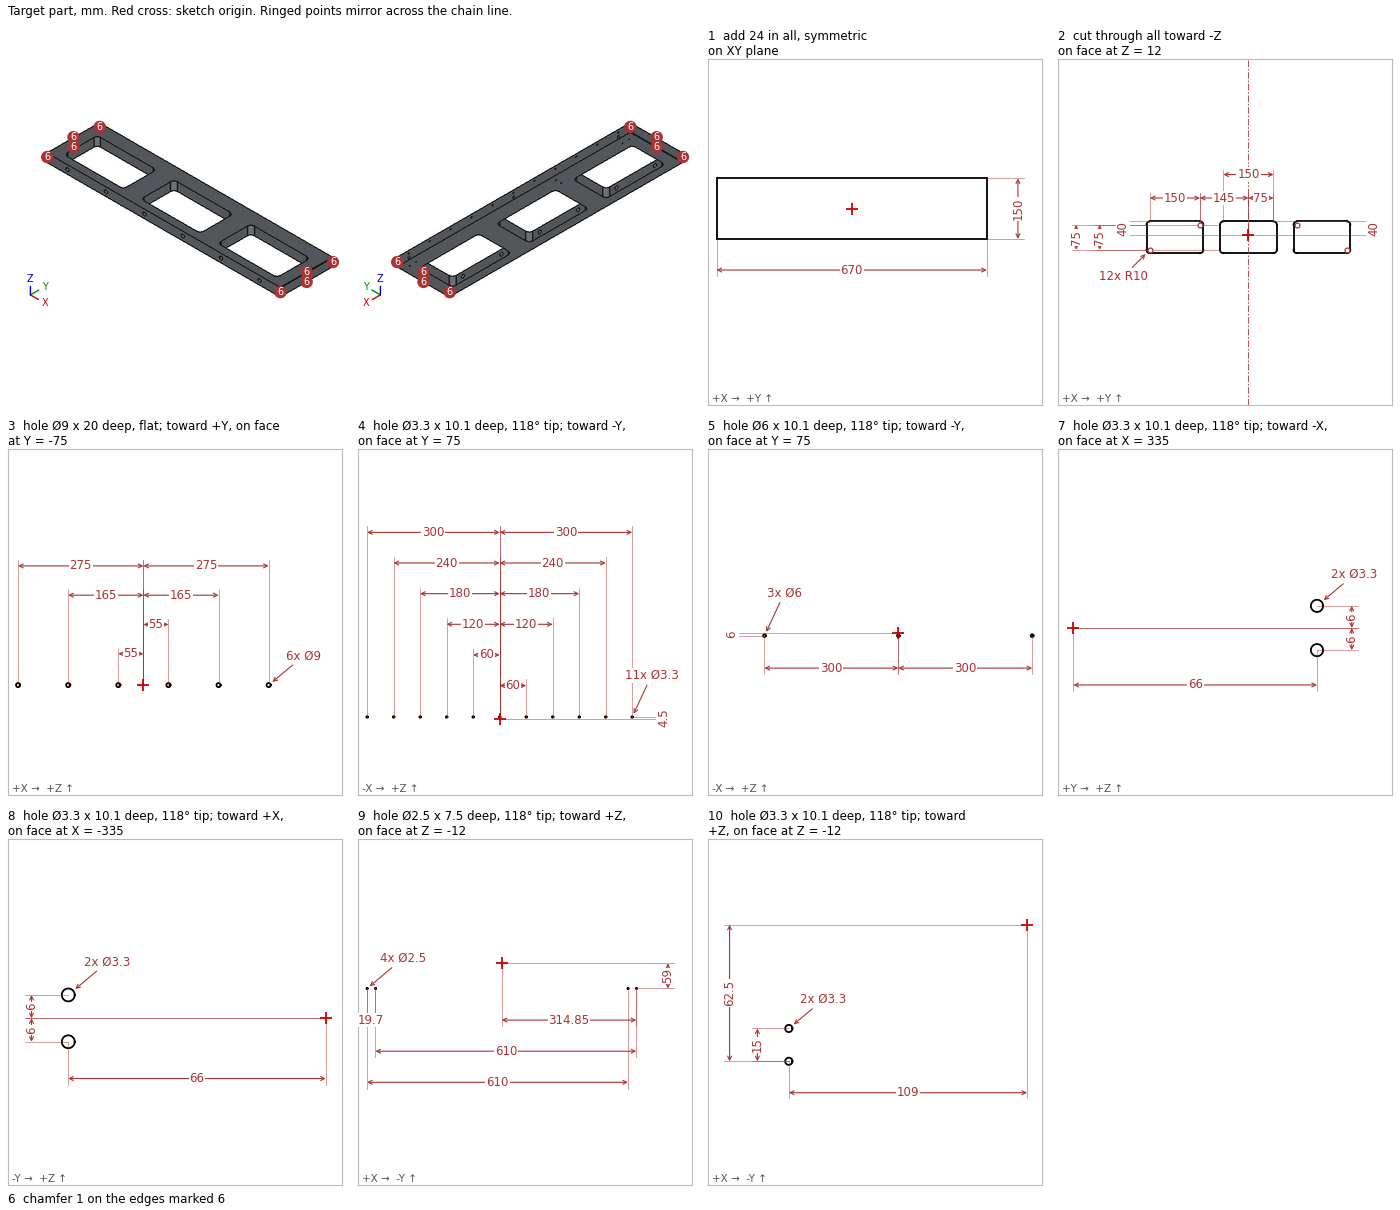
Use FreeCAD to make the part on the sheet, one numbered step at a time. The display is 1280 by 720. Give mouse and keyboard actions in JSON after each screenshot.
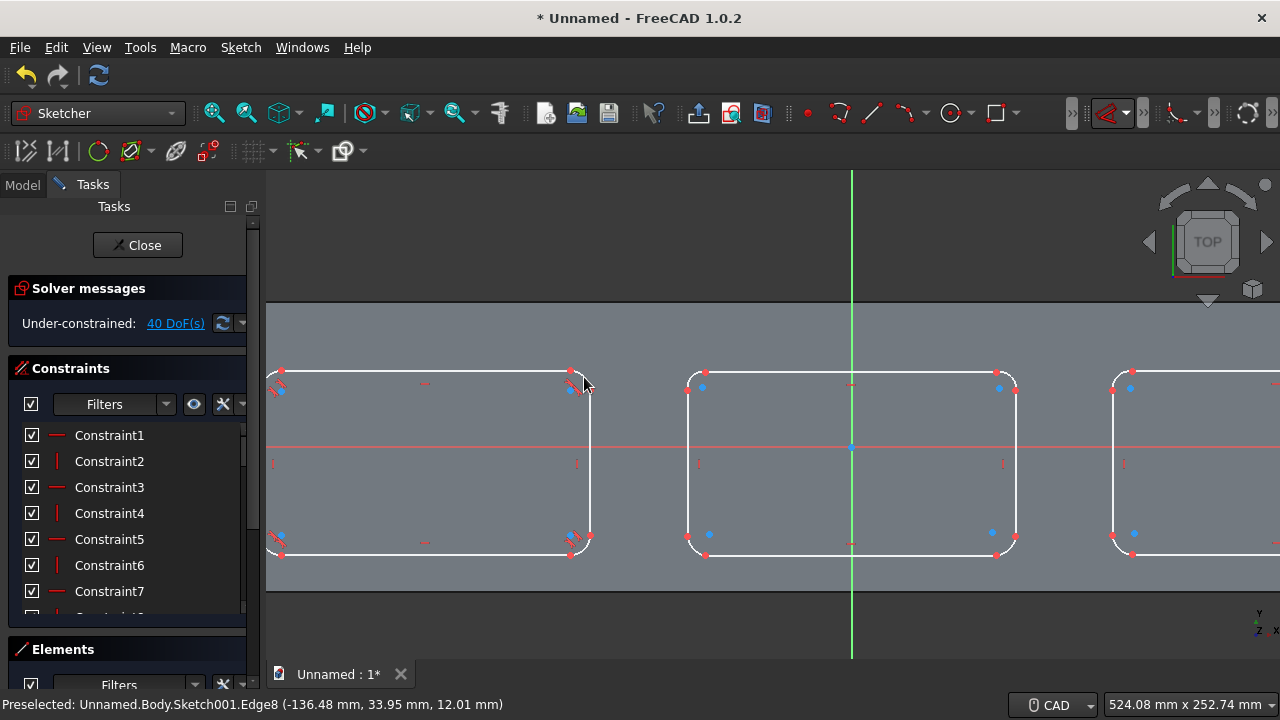
{"action": "left_click", "coordinate": [909, 372]}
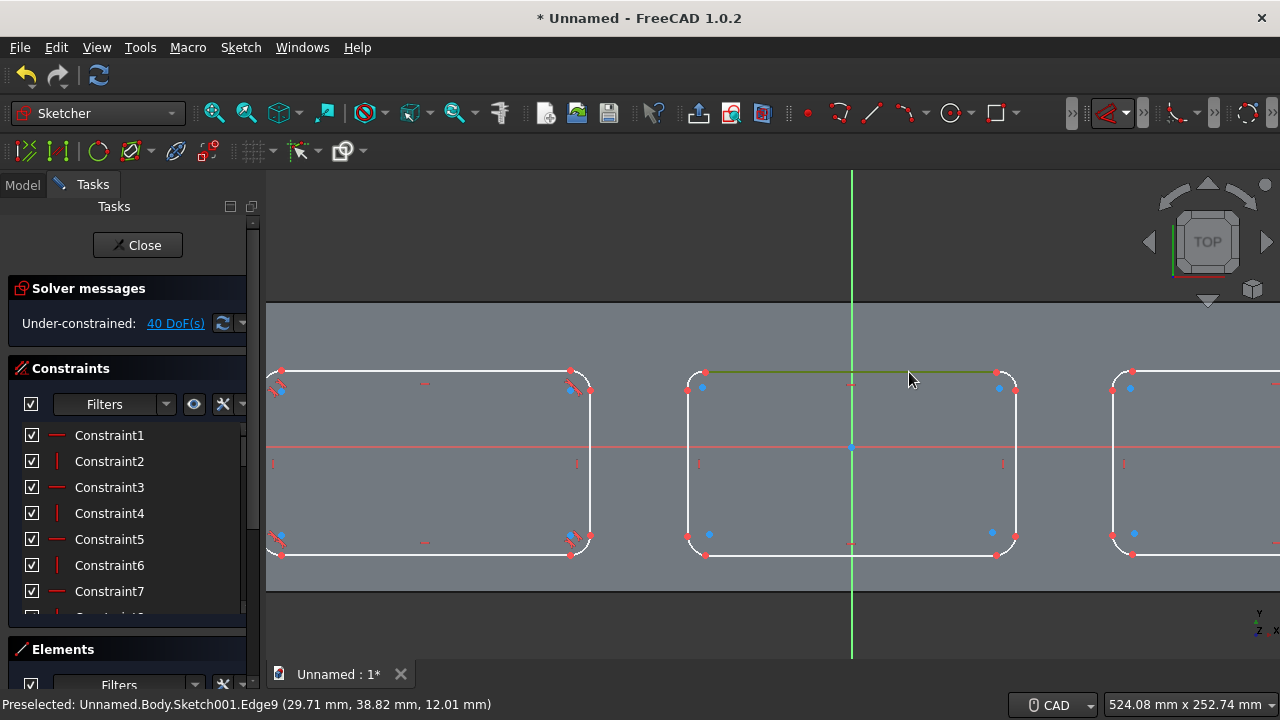
{"action": "left_click", "coordinate": [692, 377]}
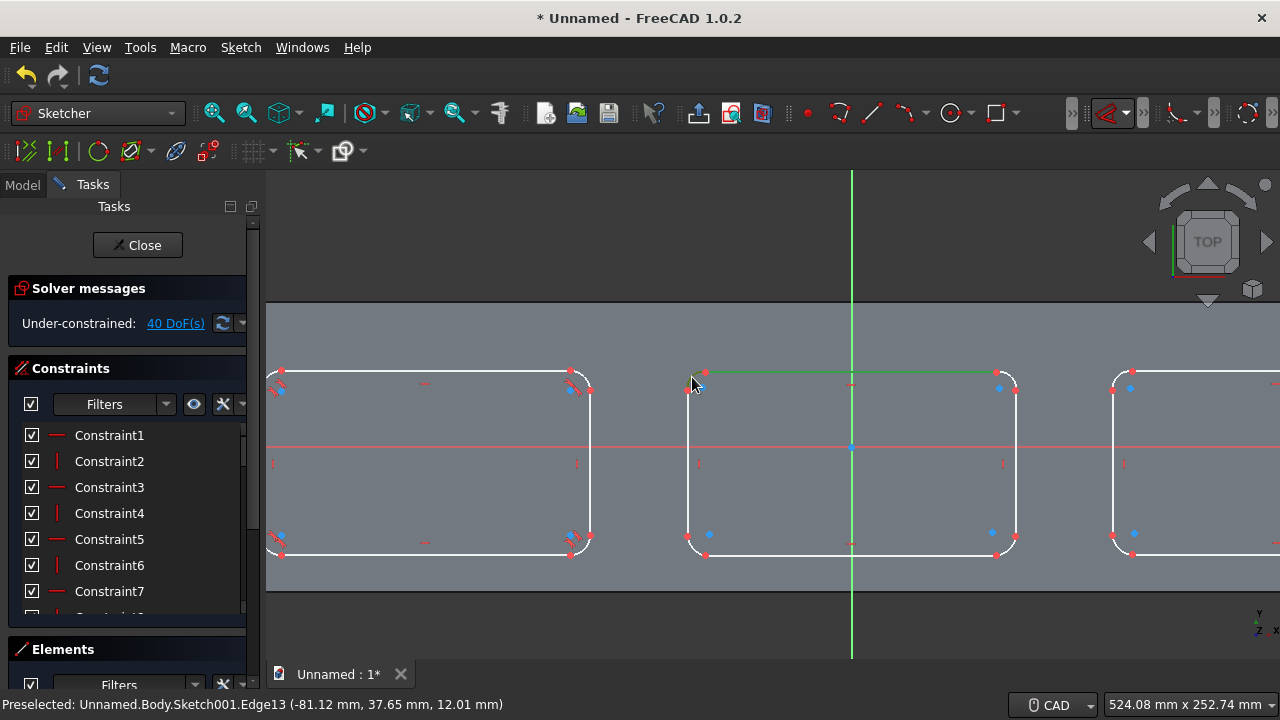
{"action": "key", "text": "t"}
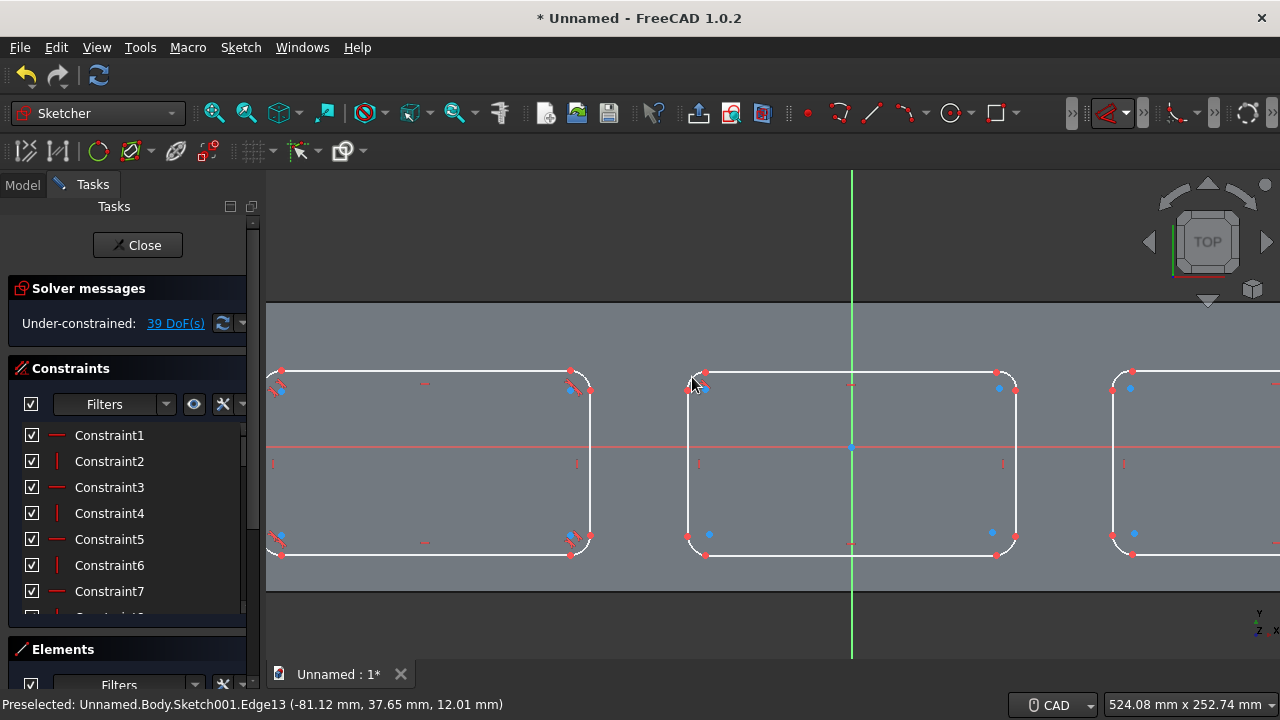
{"action": "left_click", "coordinate": [909, 372]}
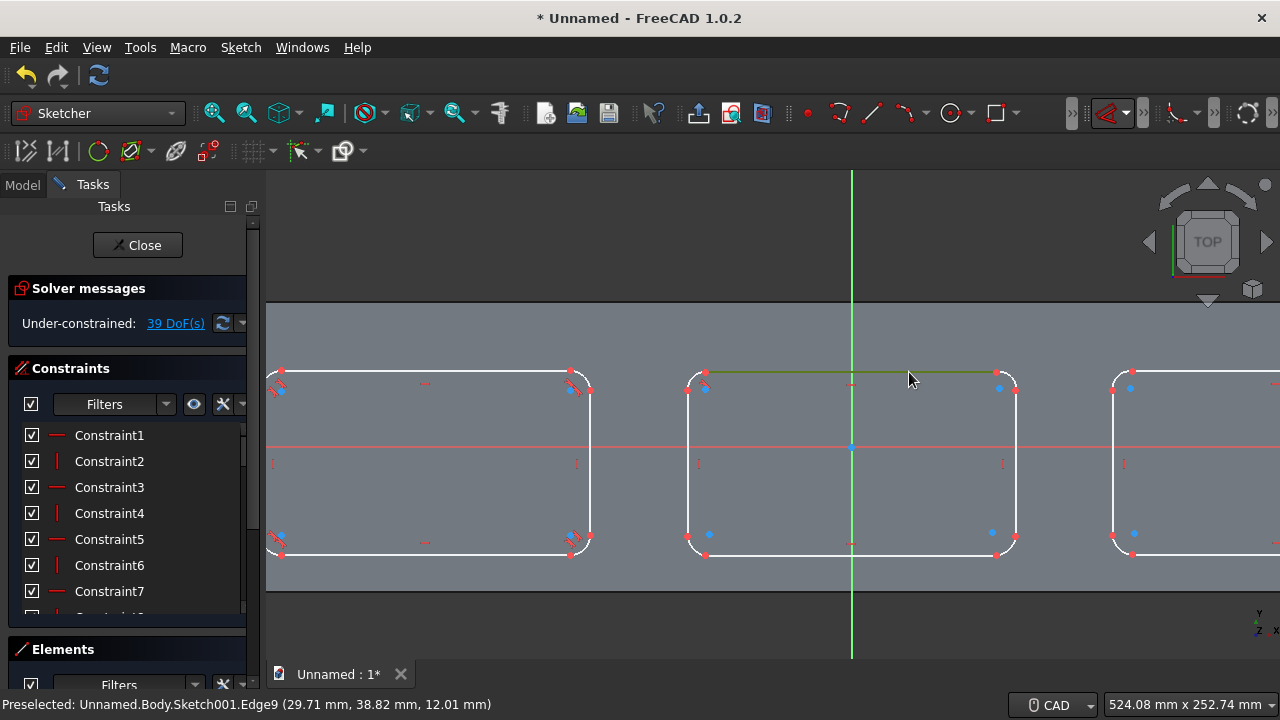
{"action": "left_click", "coordinate": [1011, 376]}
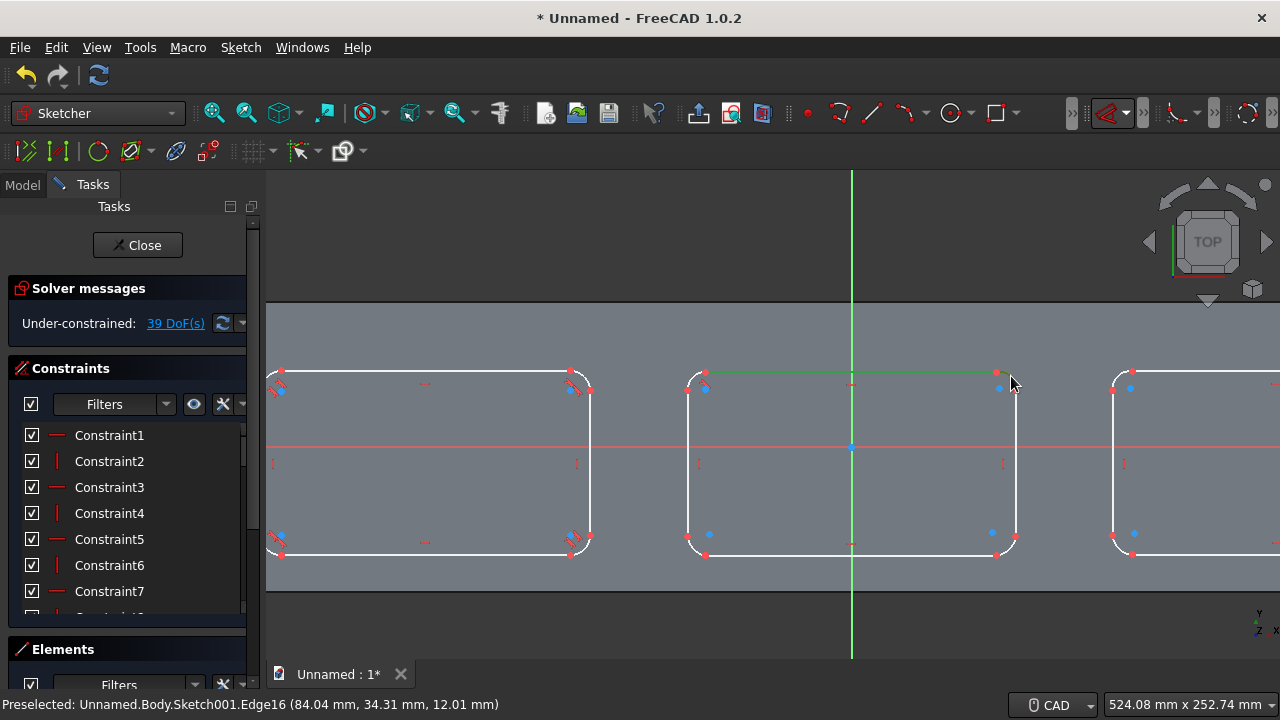
{"action": "key", "text": "t"}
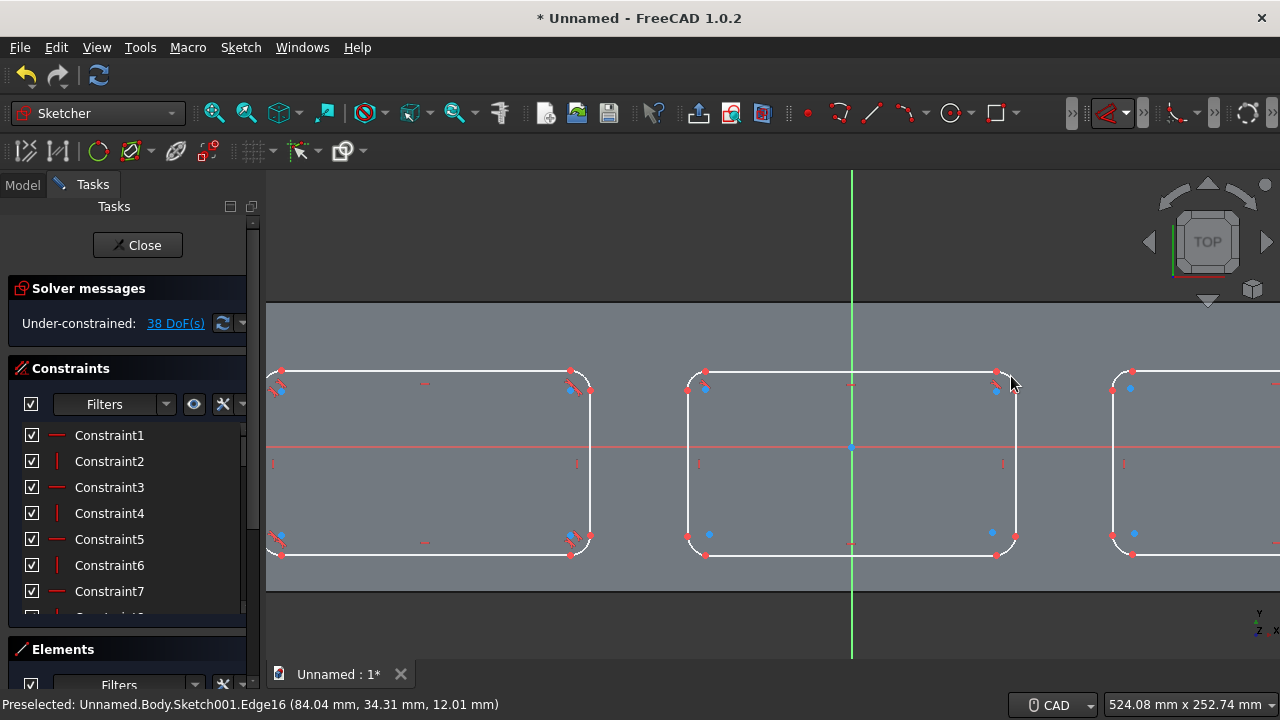
{"action": "left_click", "coordinate": [688, 434]}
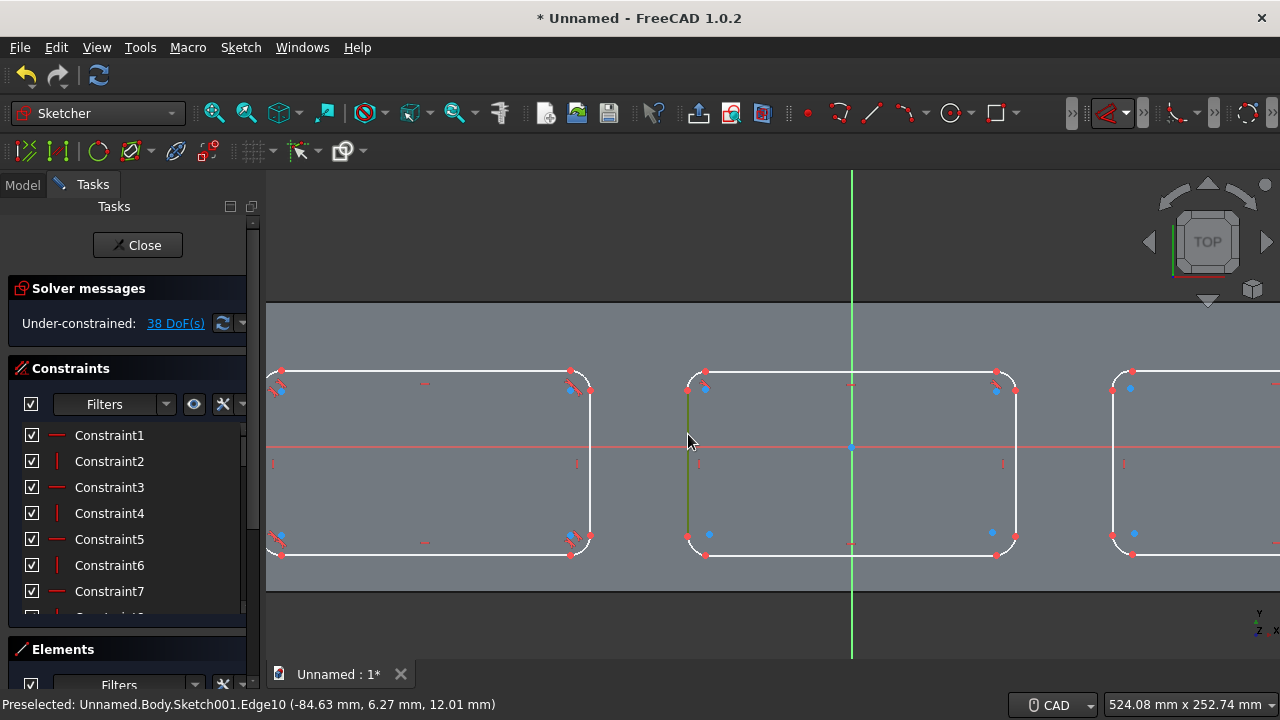
{"action": "left_click", "coordinate": [693, 377]}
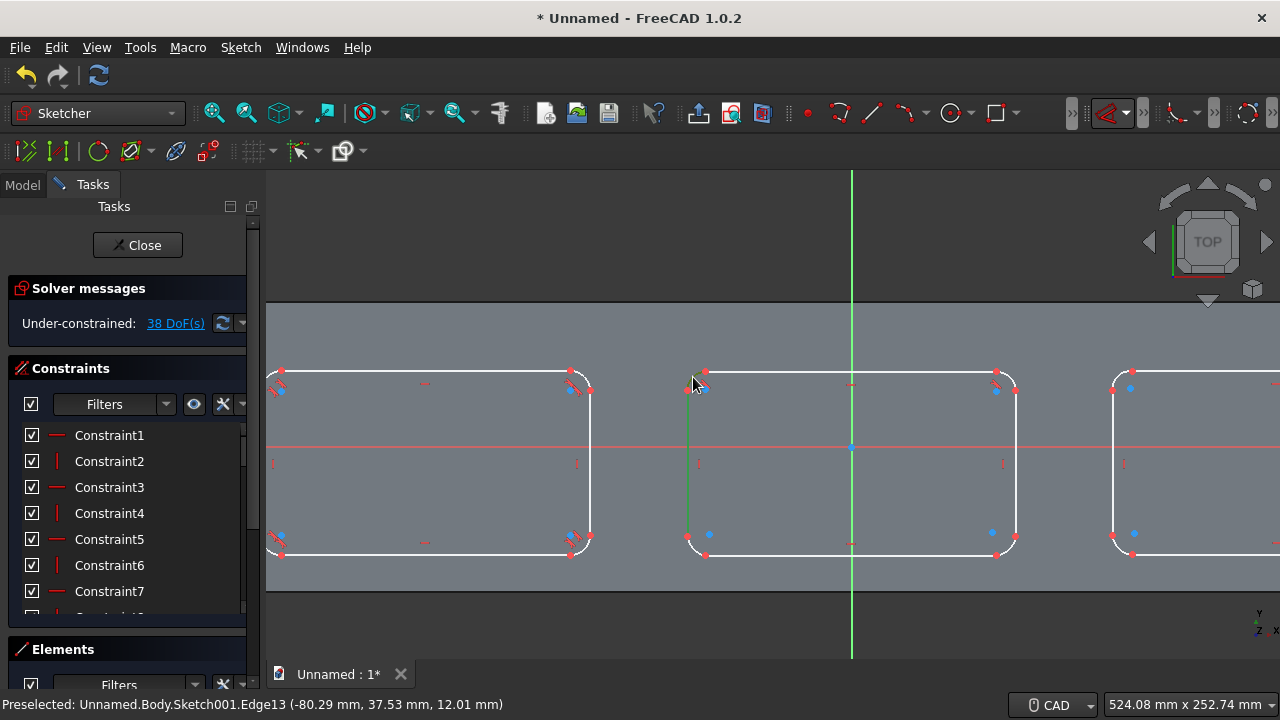
{"action": "key", "text": "t"}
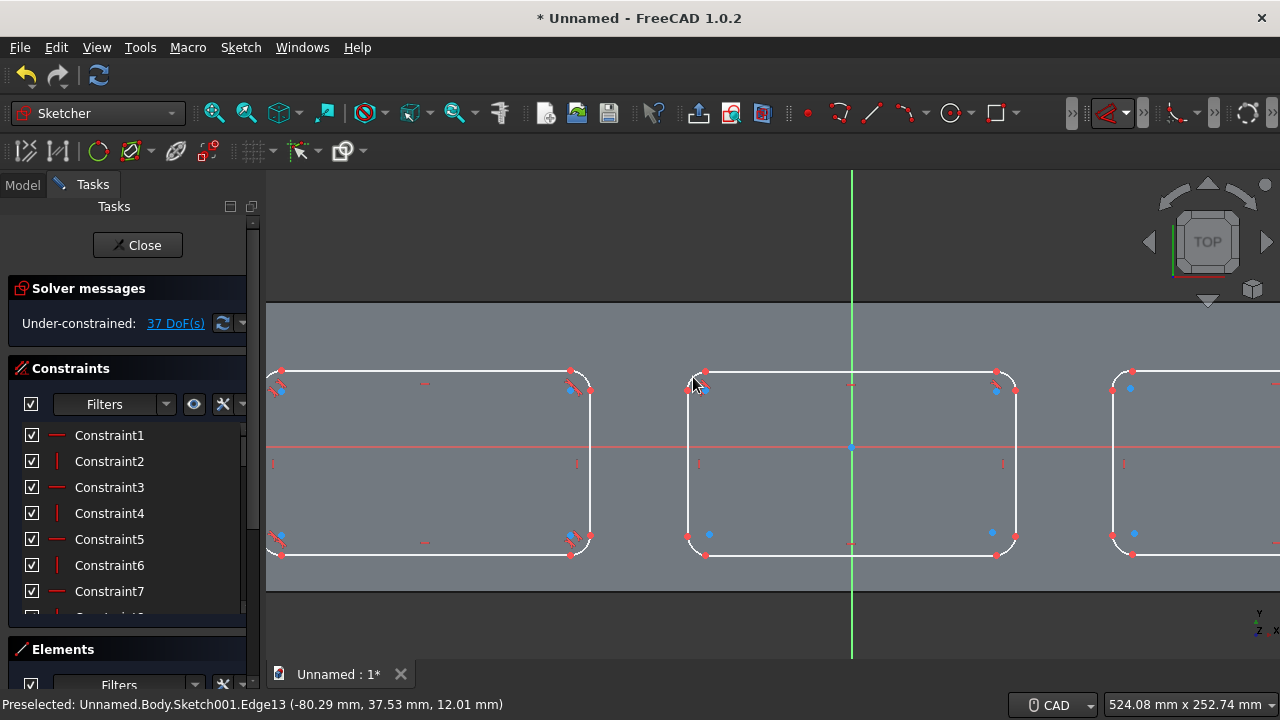
{"action": "left_click", "coordinate": [688, 434]}